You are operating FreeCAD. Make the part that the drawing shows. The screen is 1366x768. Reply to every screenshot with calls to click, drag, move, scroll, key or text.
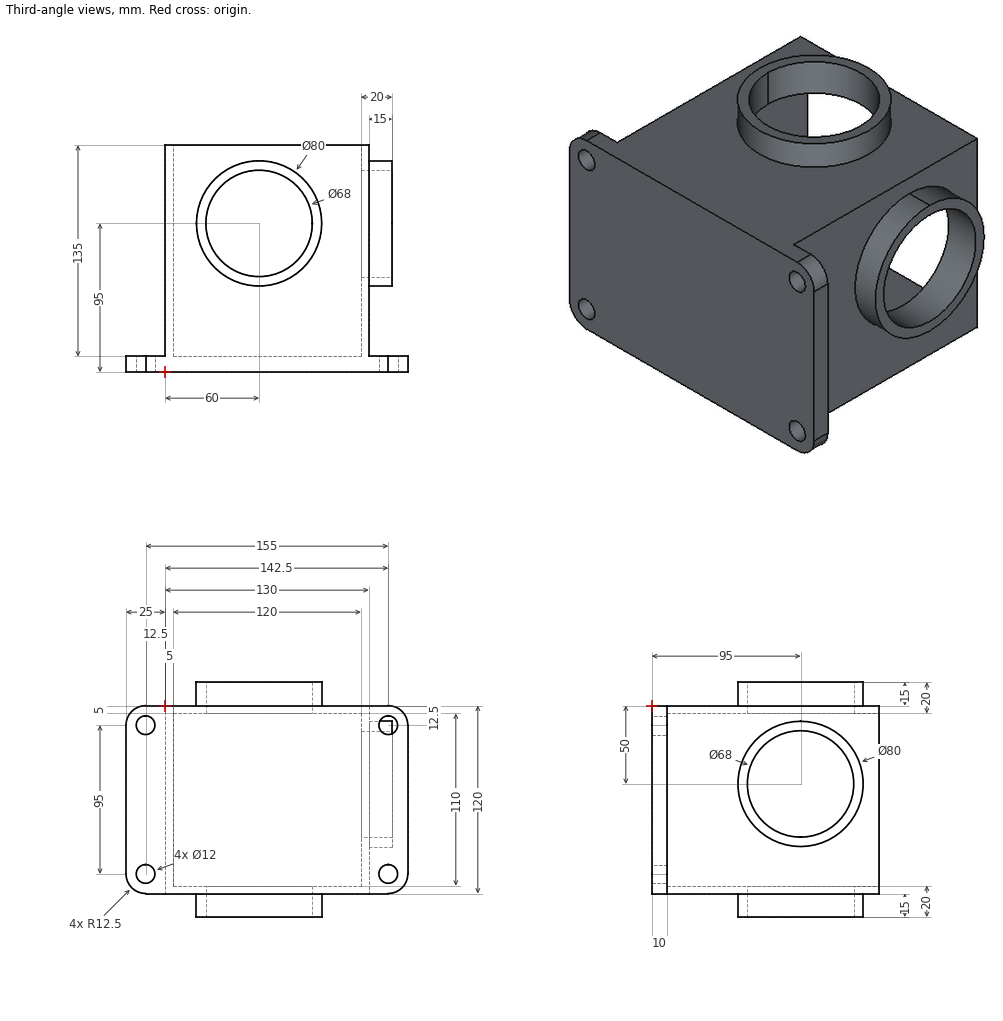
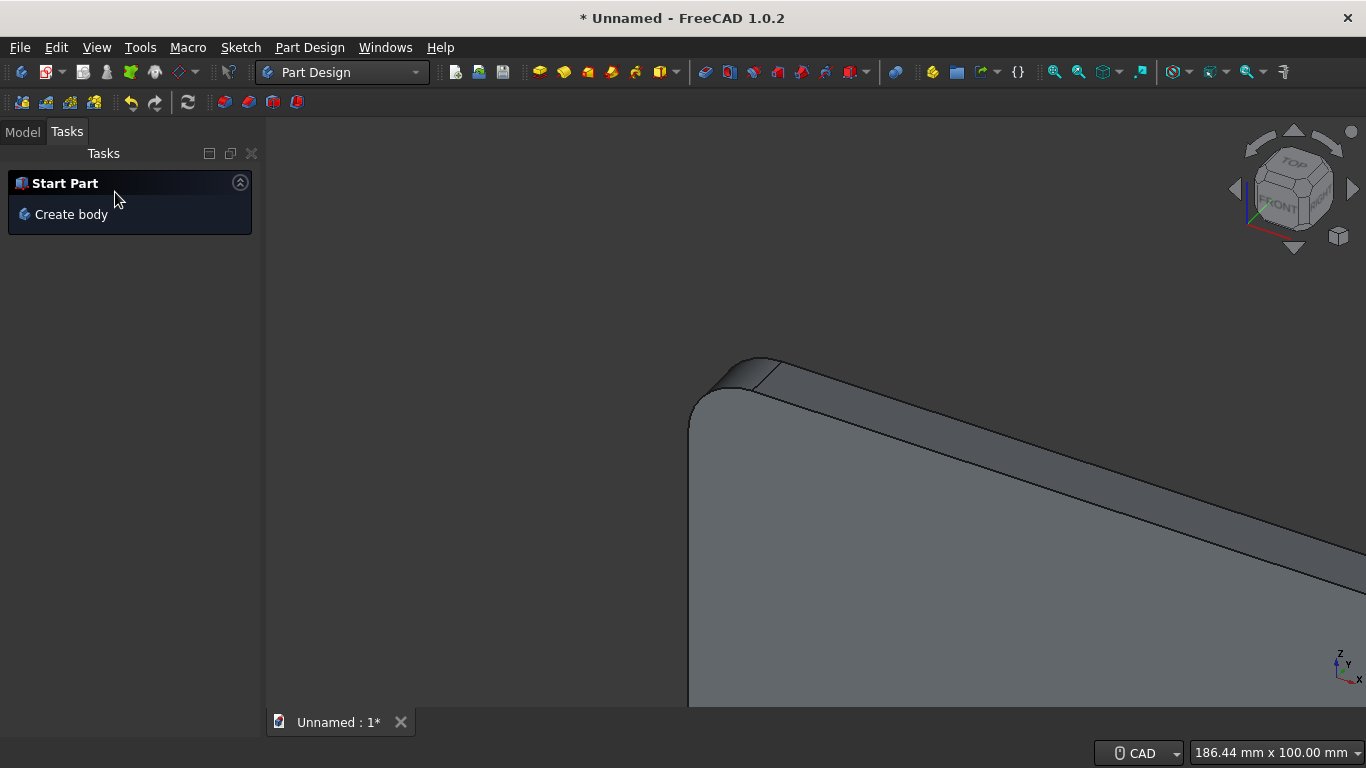
click(1056, 72)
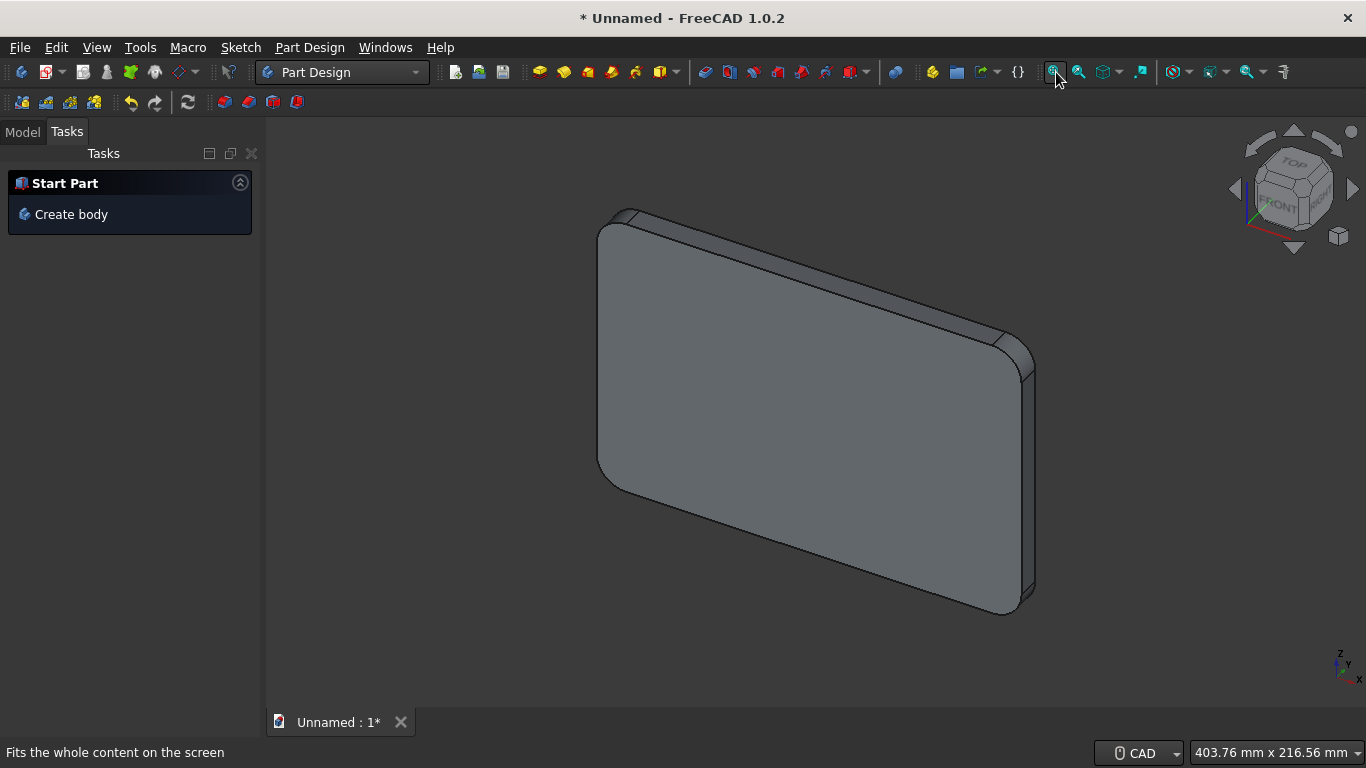
key(4)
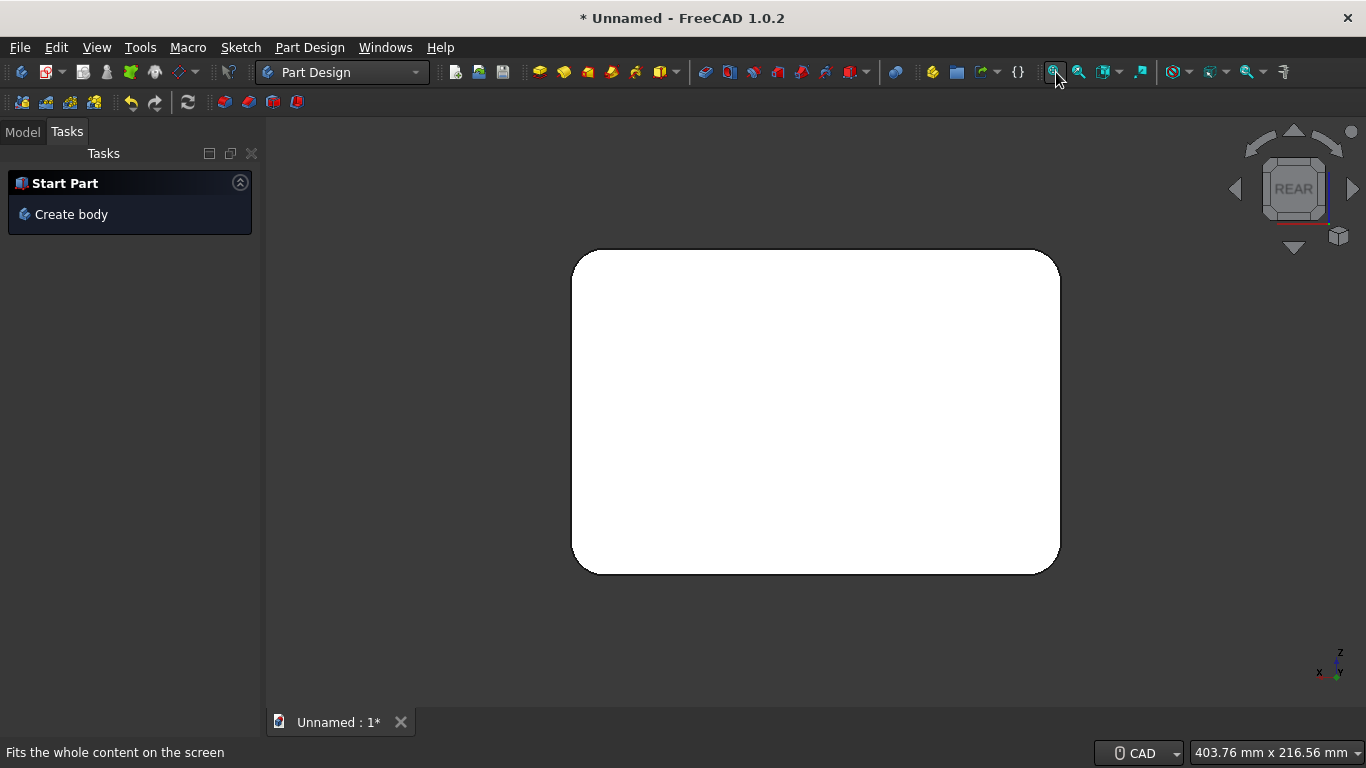
click(746, 411)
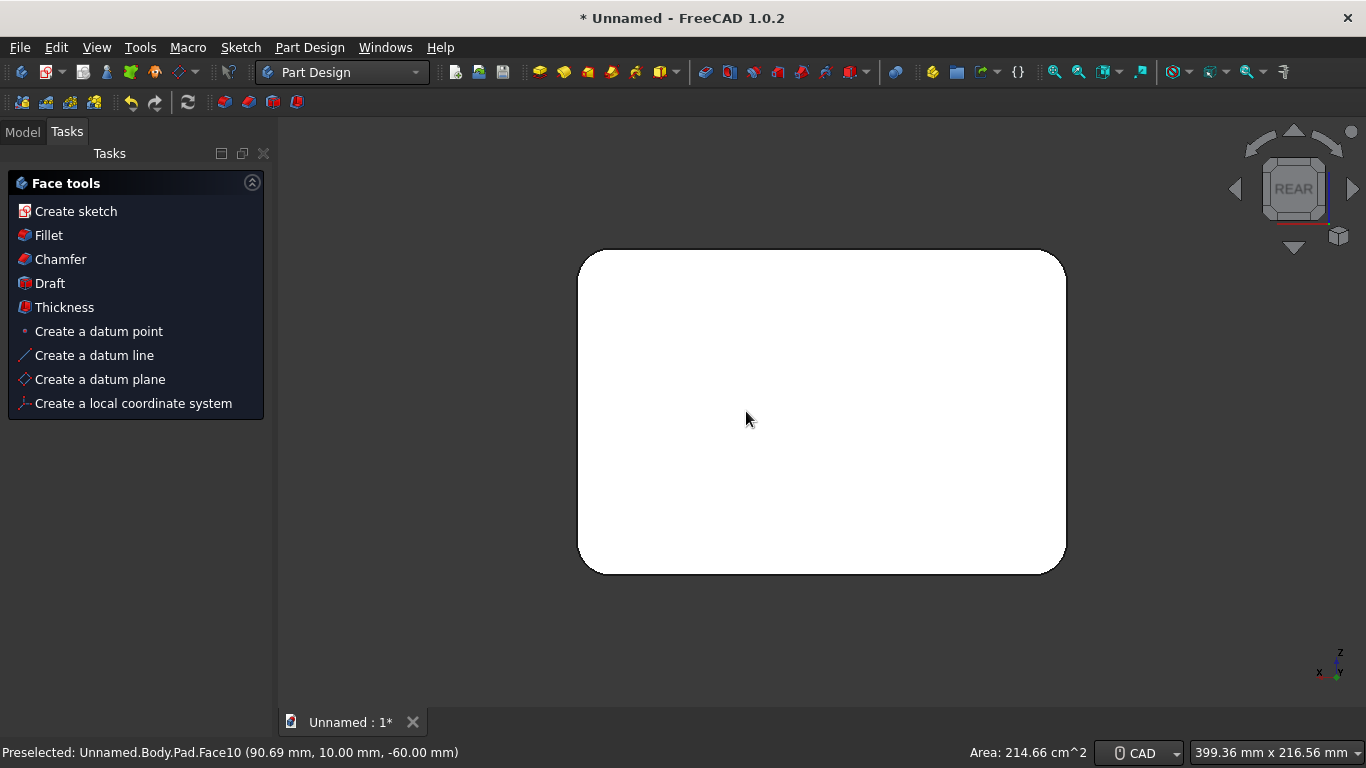
click(46, 72)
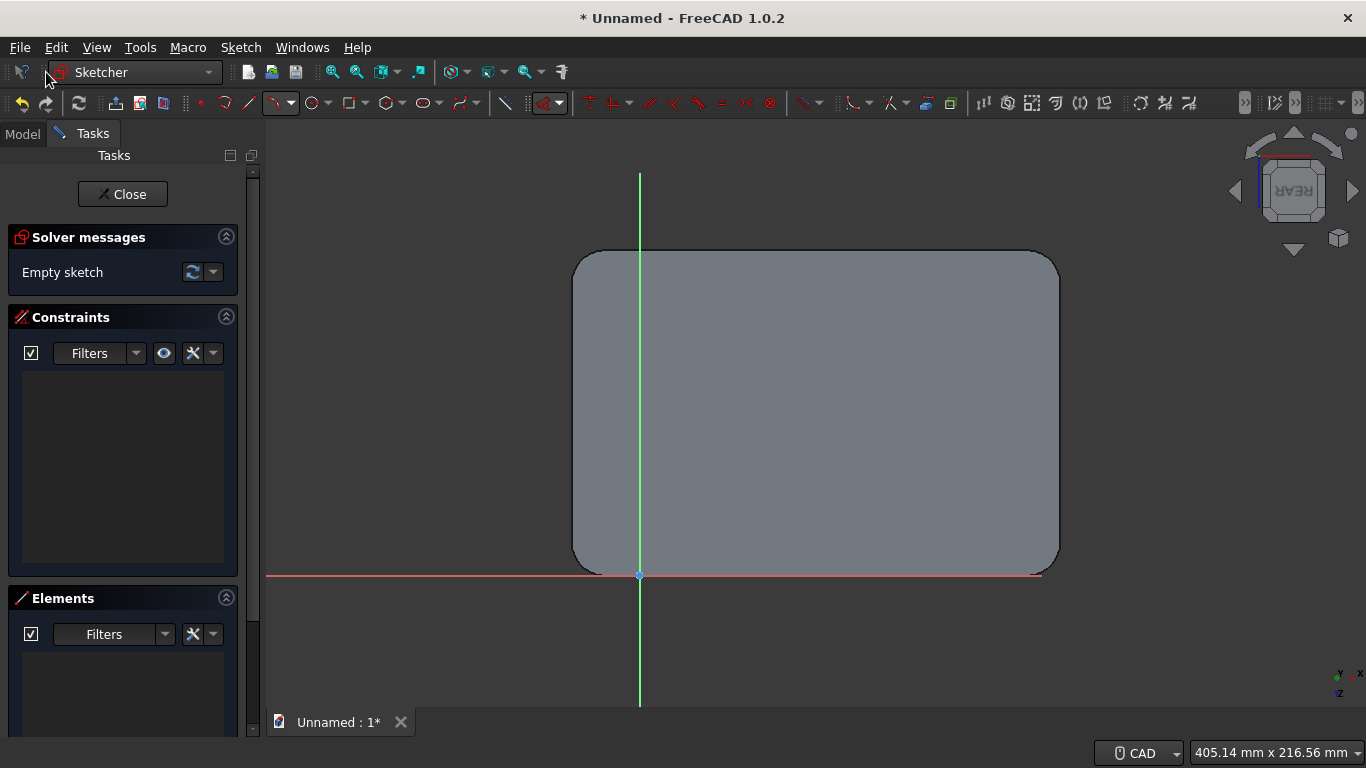
click(312, 104)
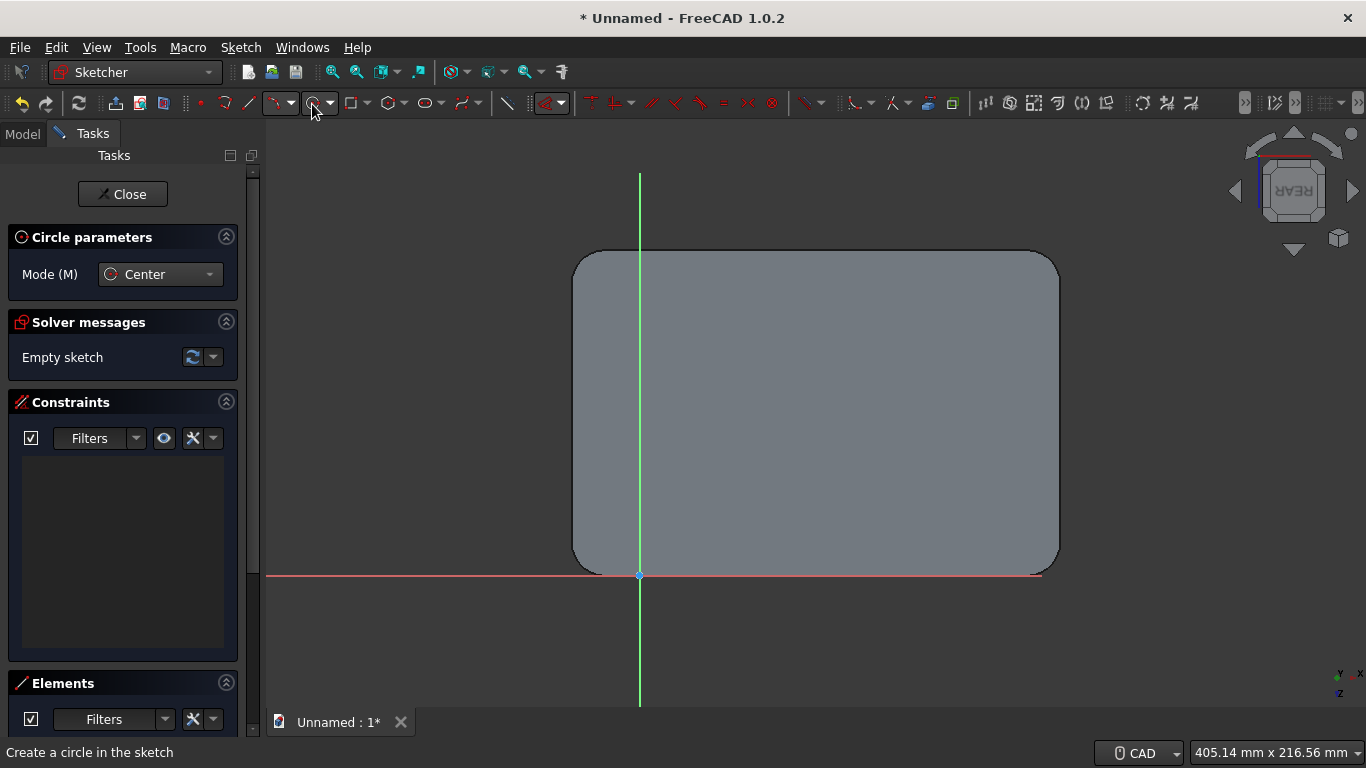
scroll(606, 284, up, 2)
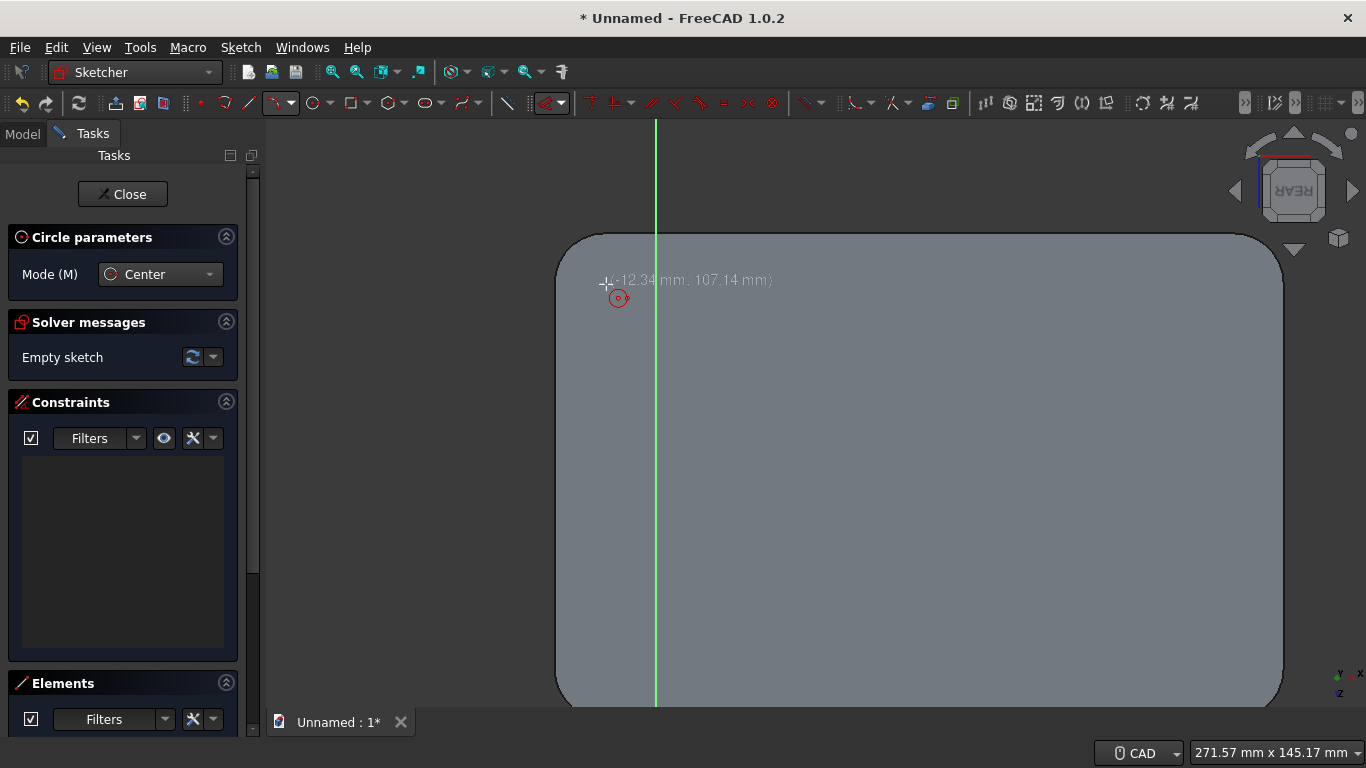
click(605, 284)
move(622, 267)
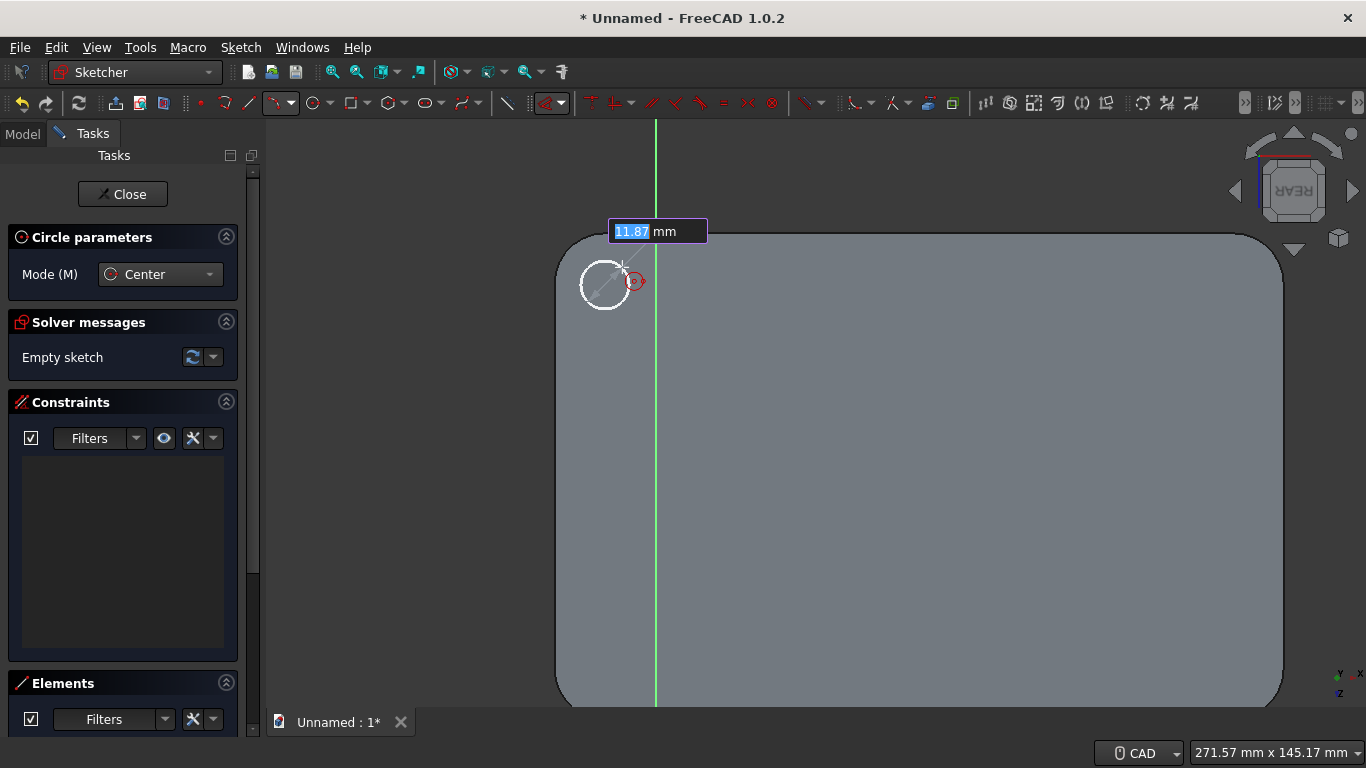
text(12)
key(Return)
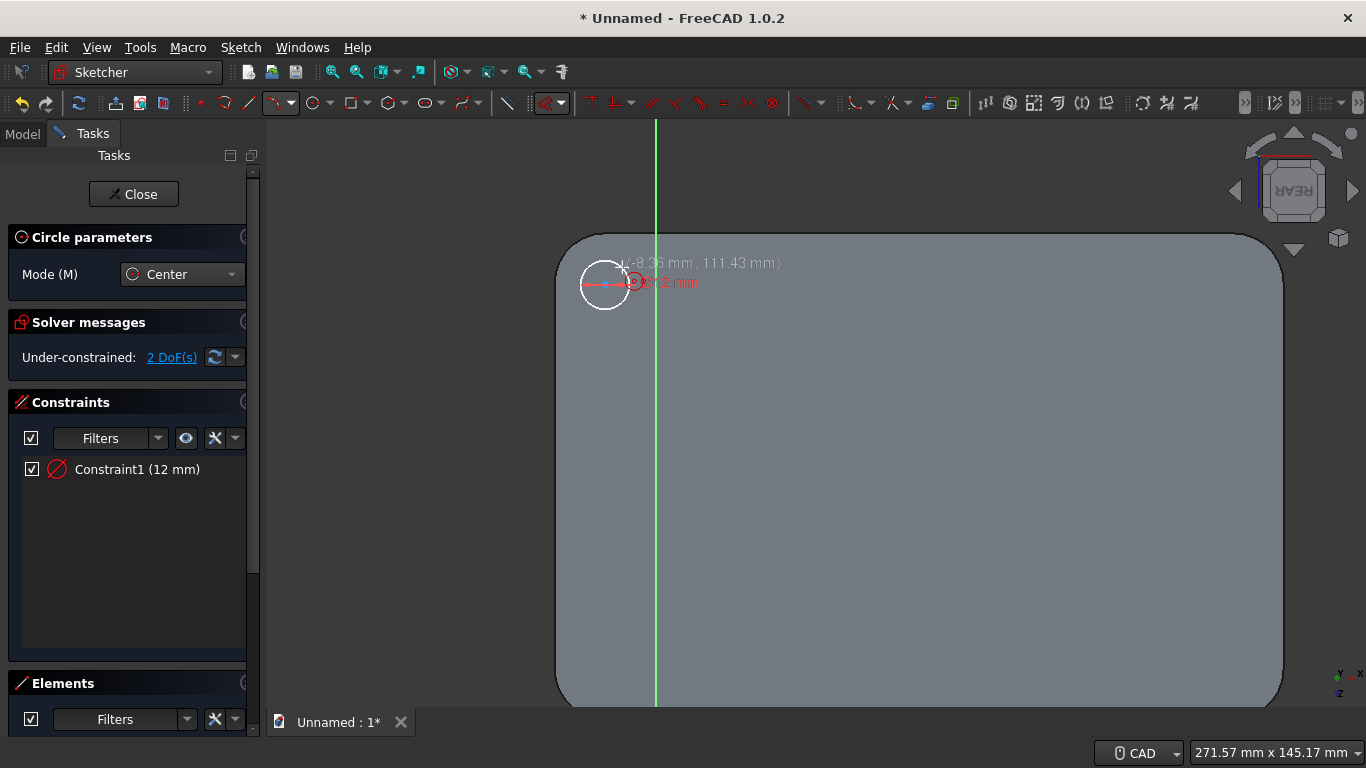
scroll(294, 147, down, 1)